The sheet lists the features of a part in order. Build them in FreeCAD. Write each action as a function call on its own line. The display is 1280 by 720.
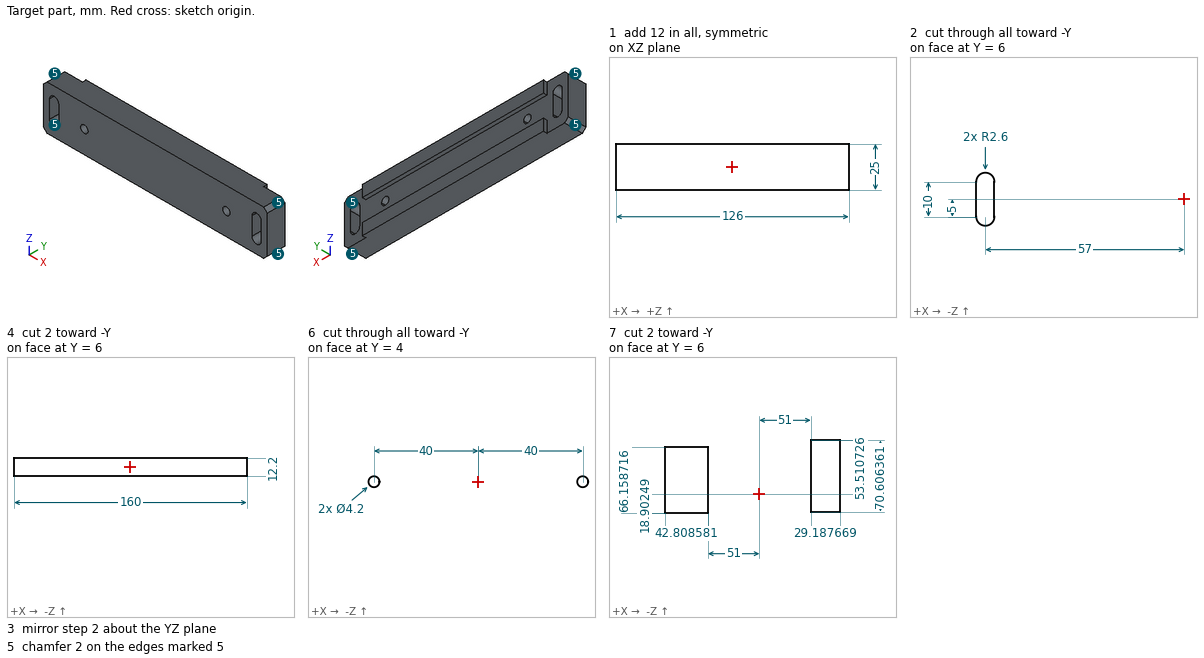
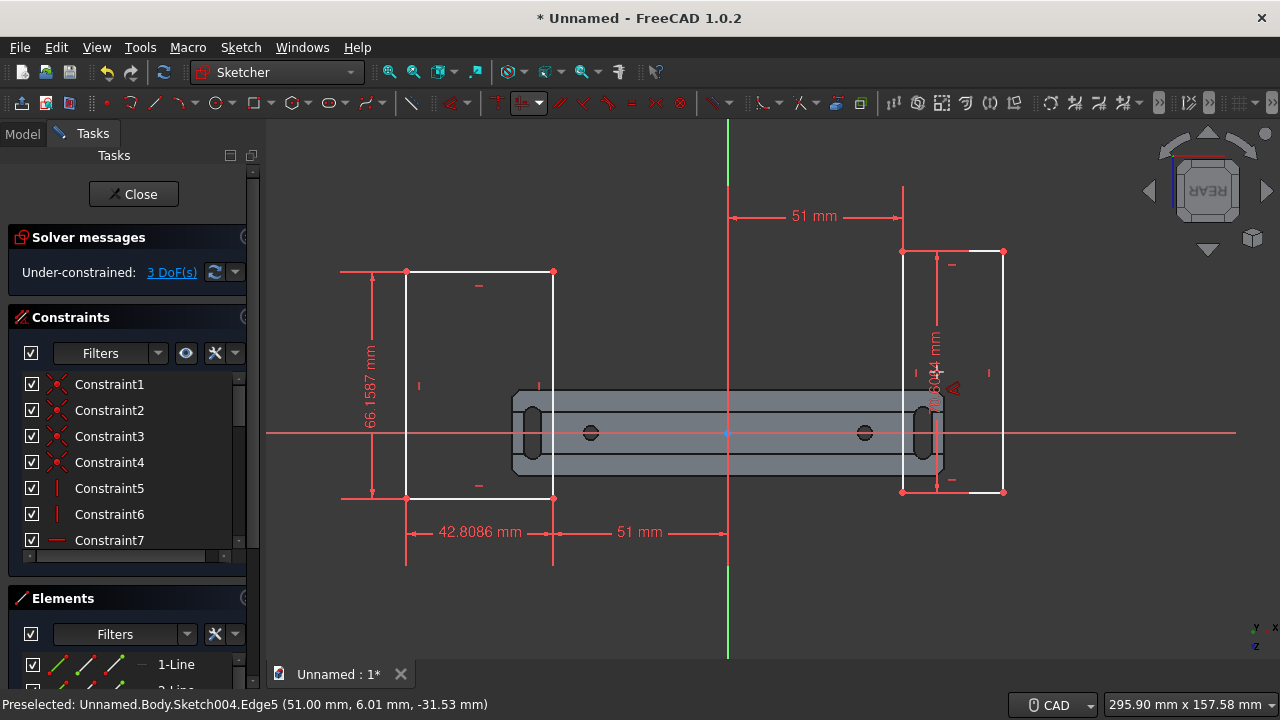
click(933, 493)
click(953, 527)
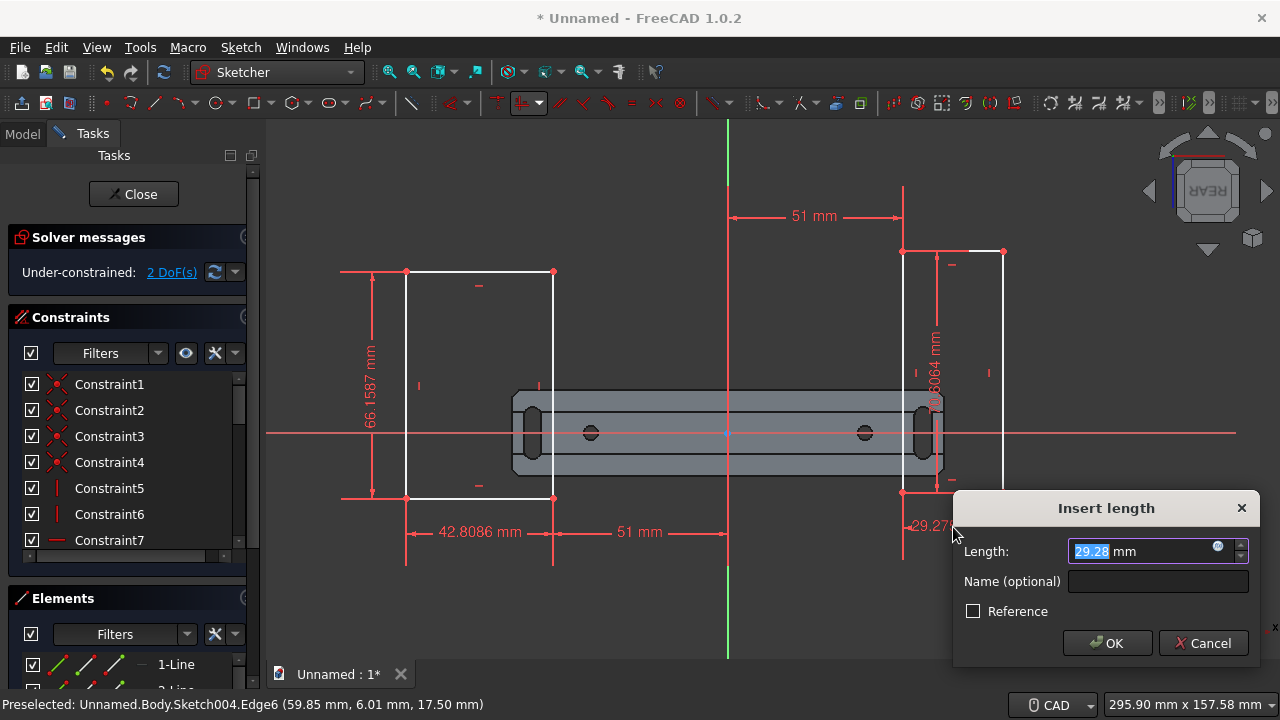
text(29.187669)
key(Return)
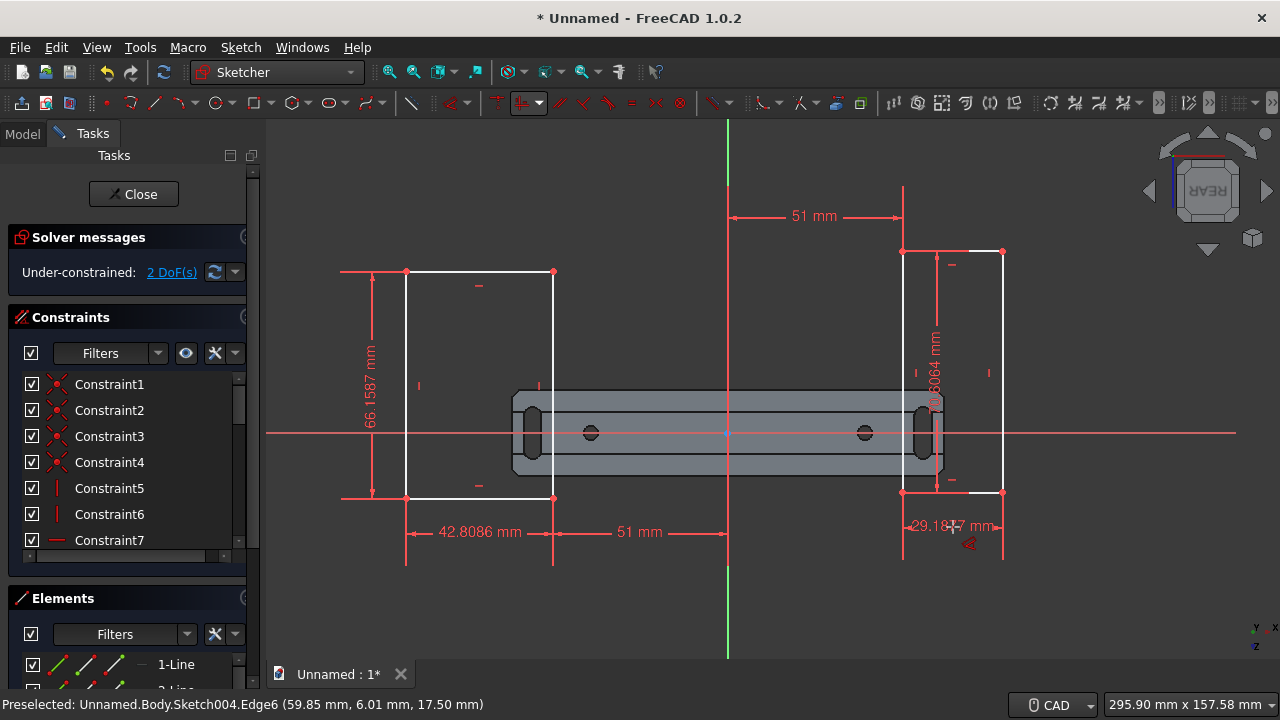
click(406, 499)
click(372, 466)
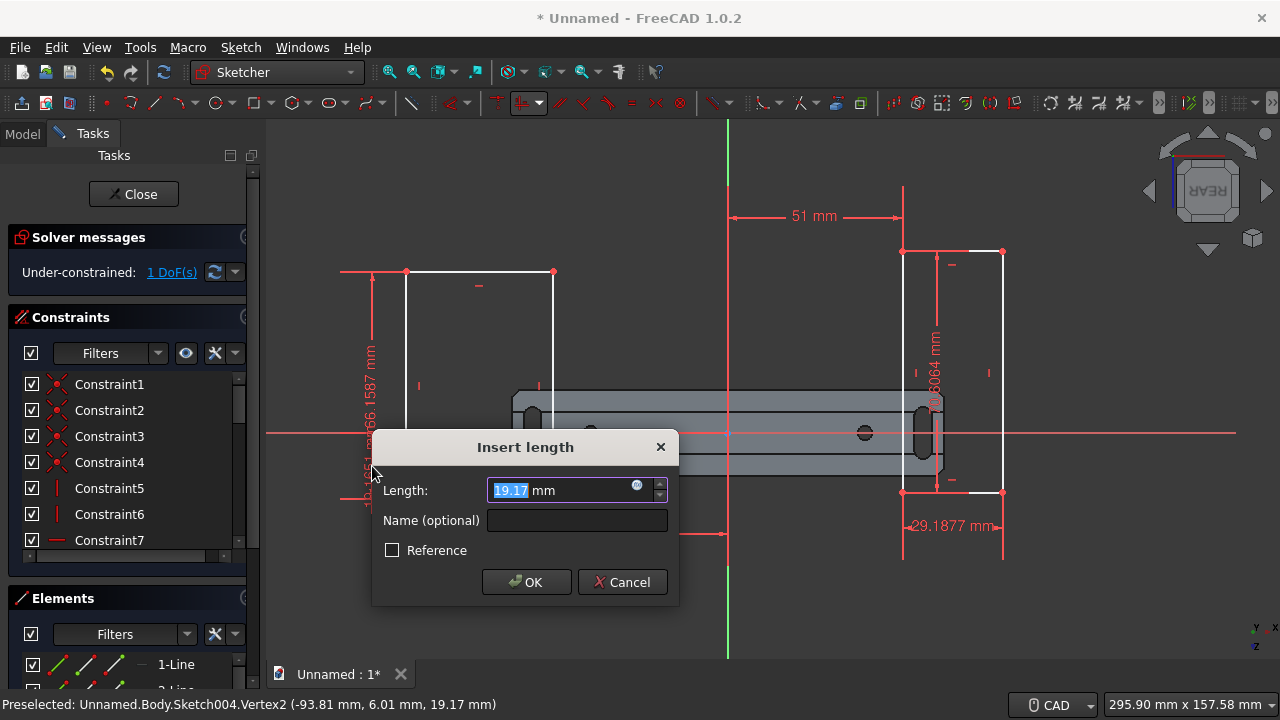
text(18.90249)
key(Return)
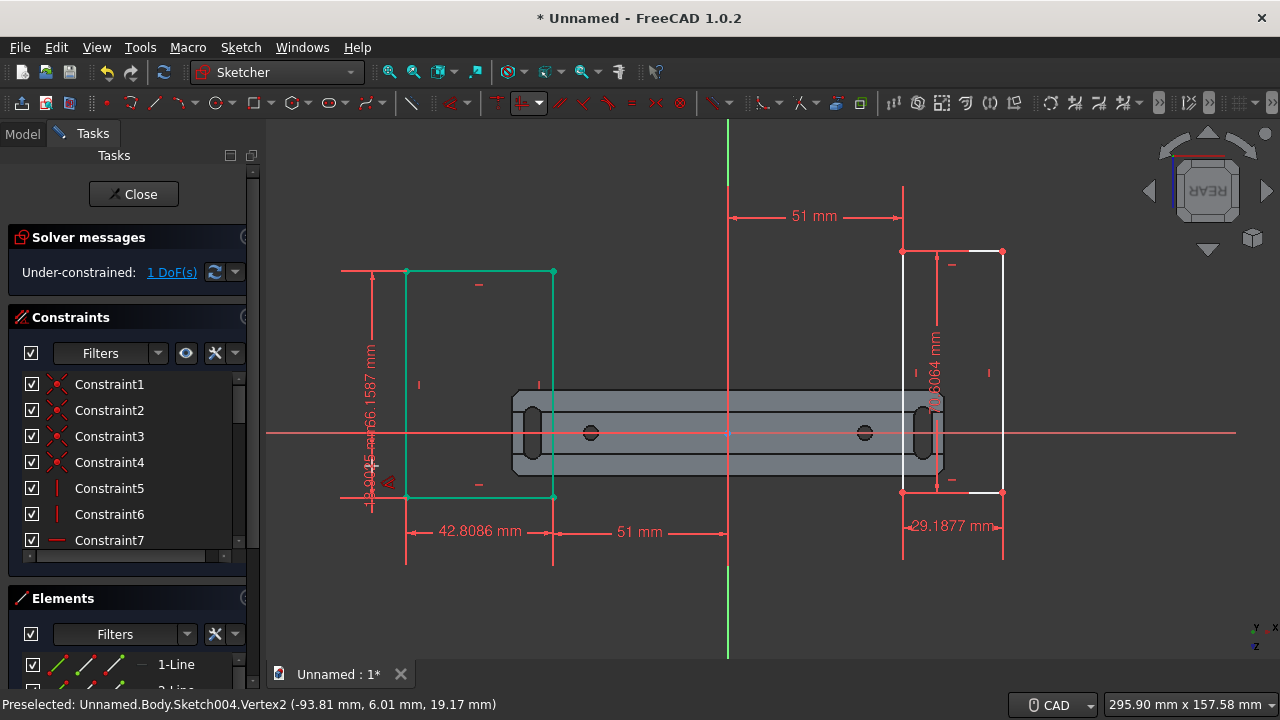
click(903, 251)
click(937, 342)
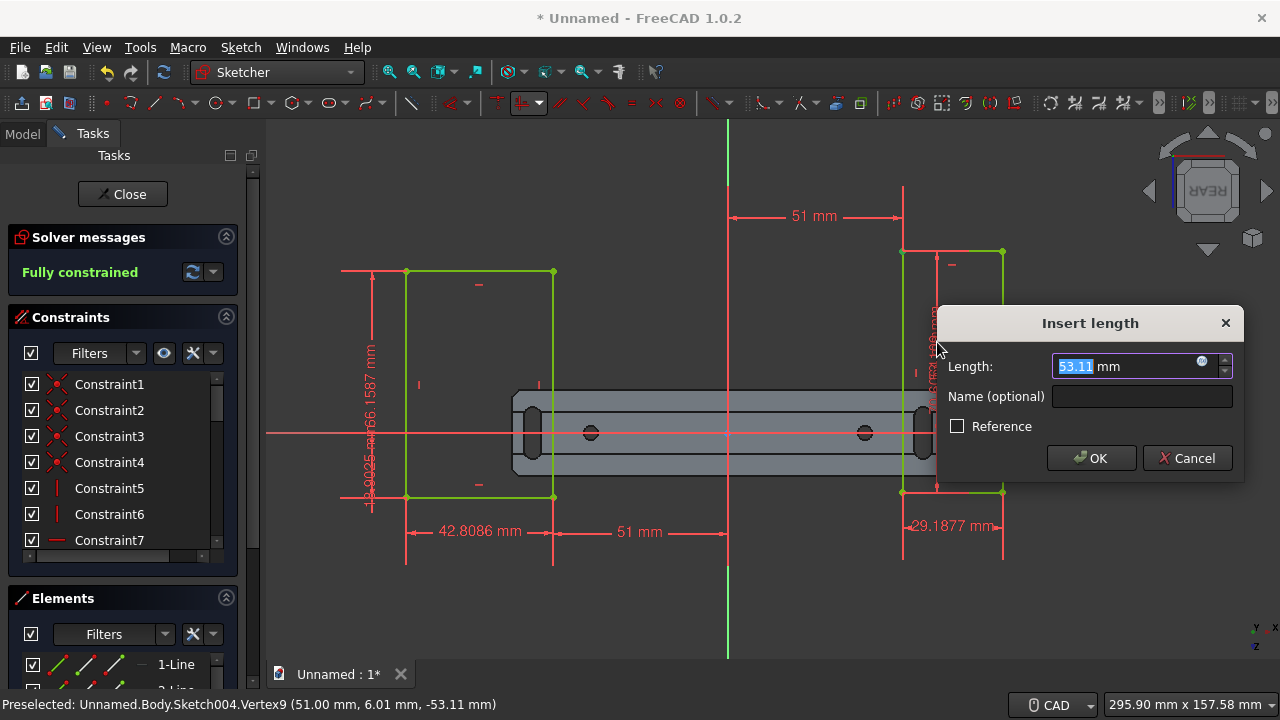
text(53.510726)
key(Return)
key(Escape)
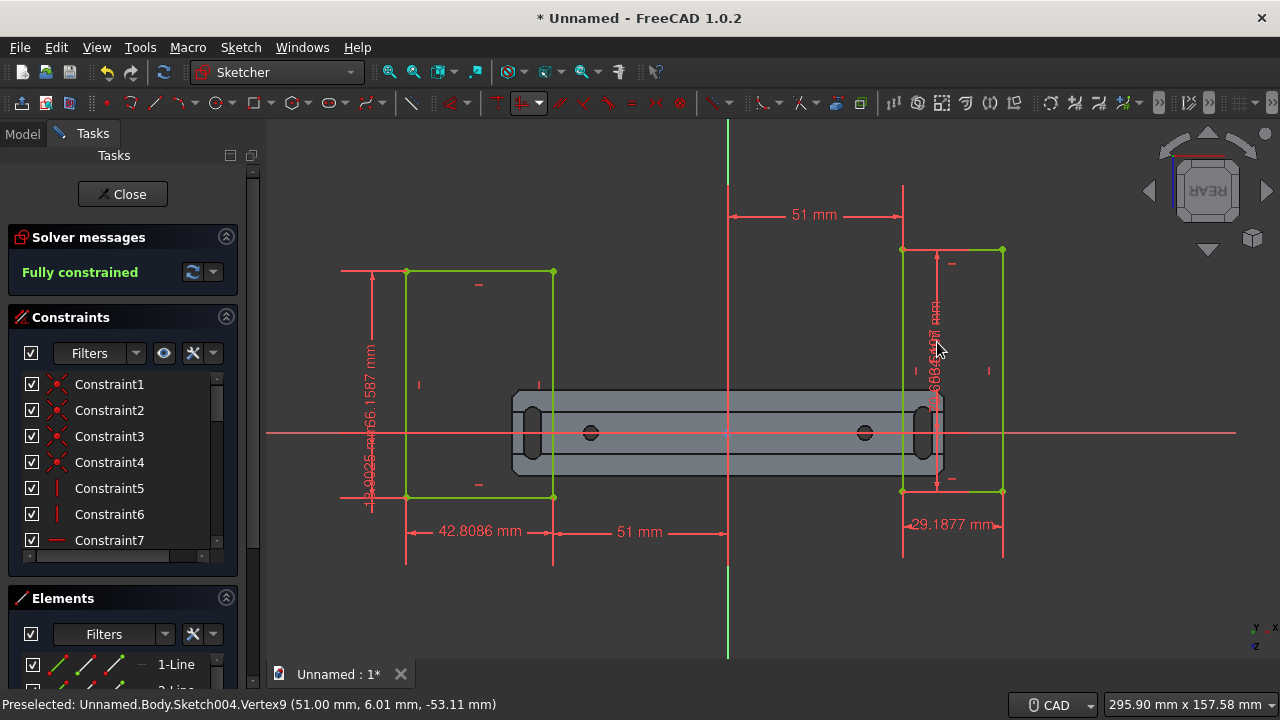
click(123, 194)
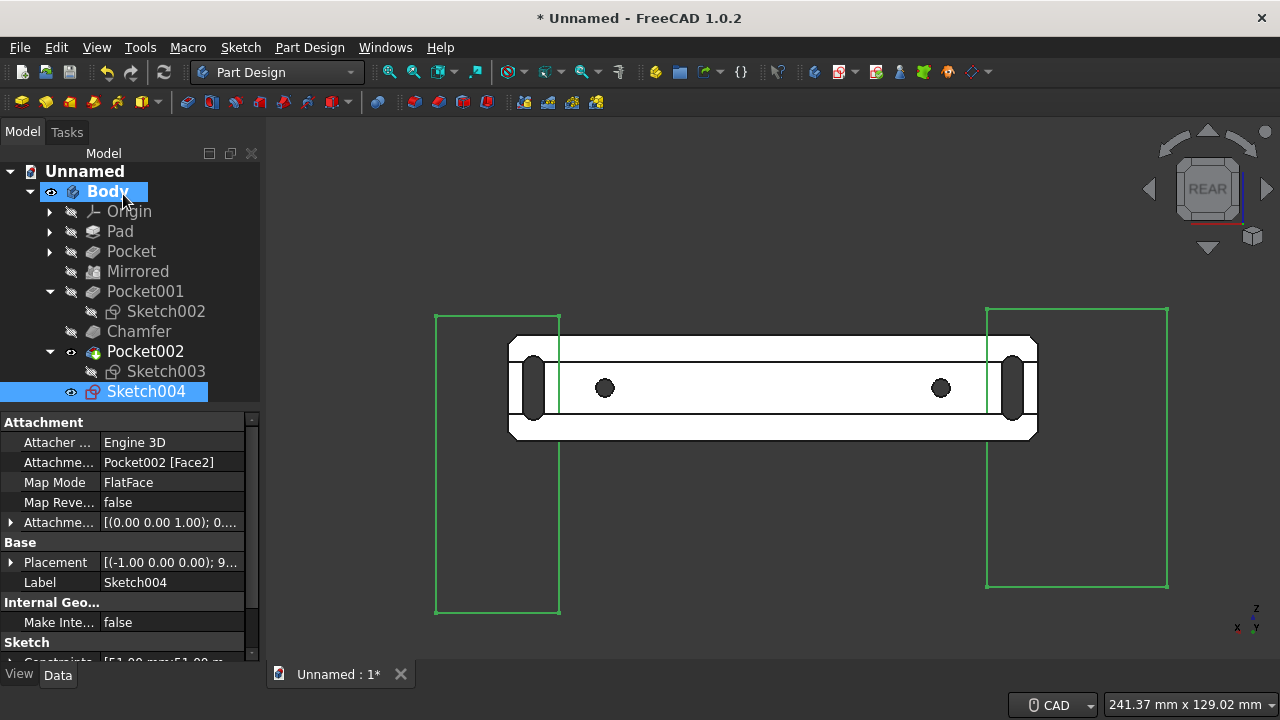
click(188, 102)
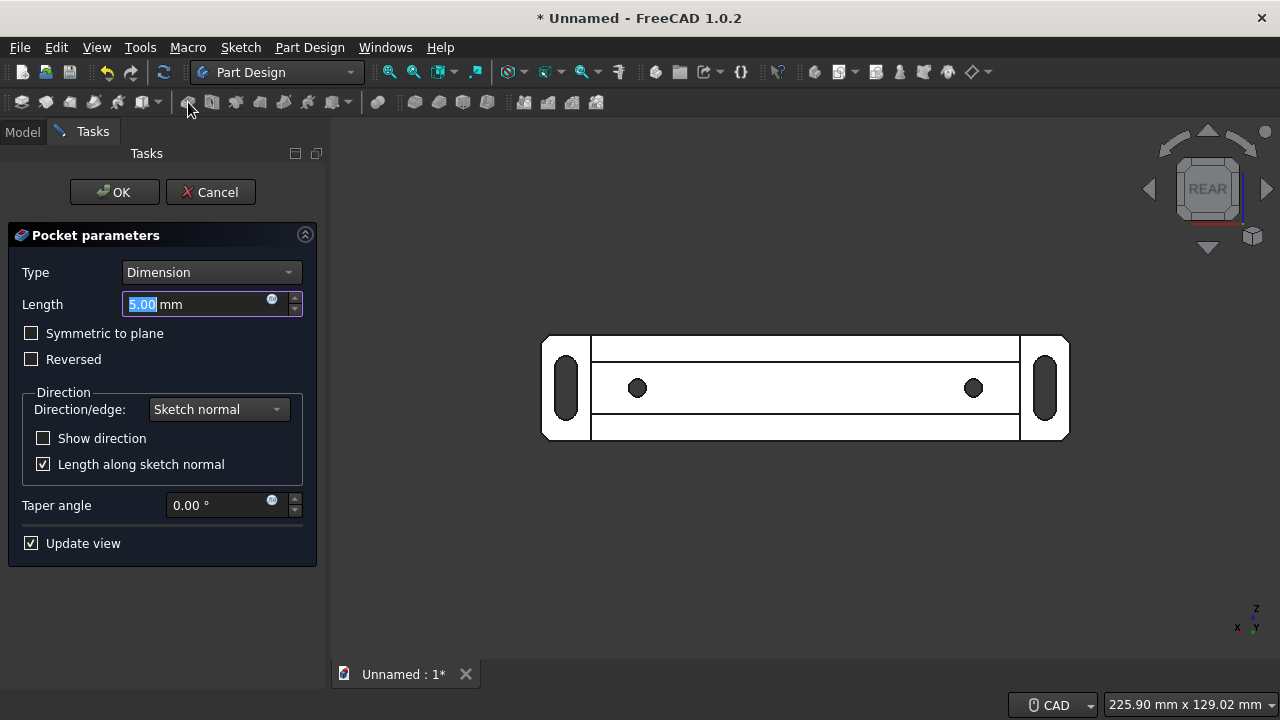
text(2)
key(Tab)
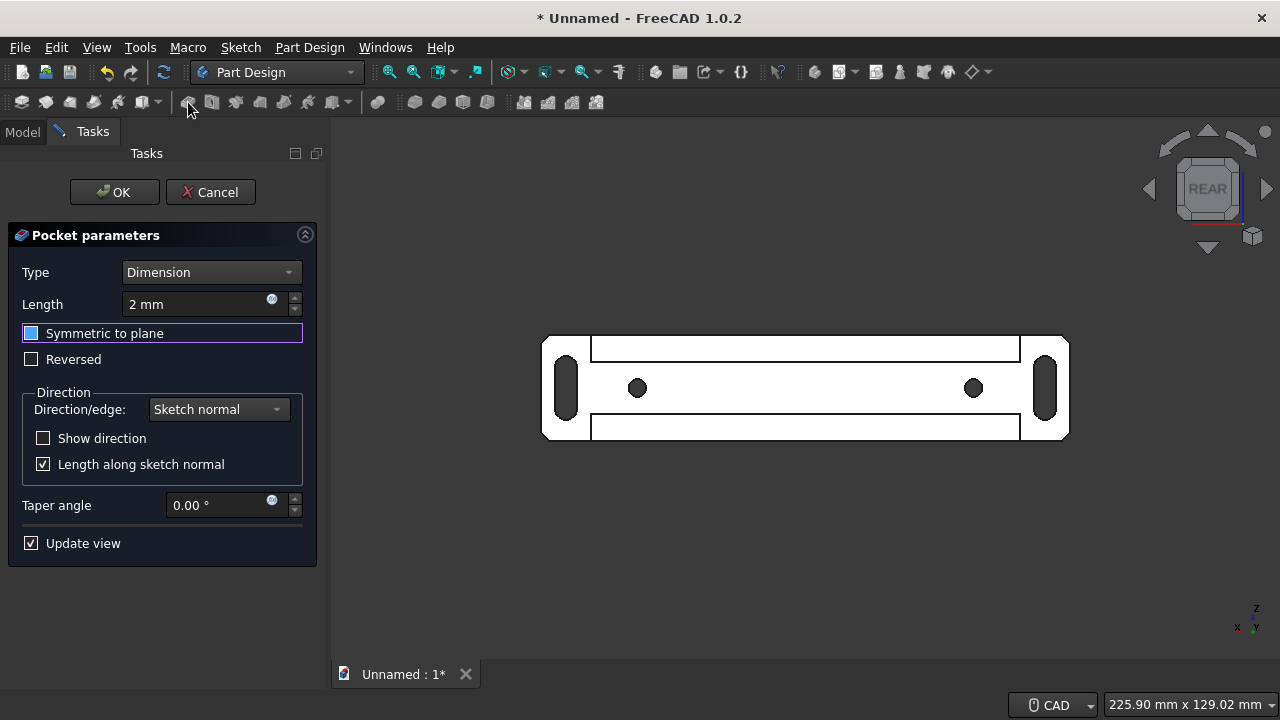
click(115, 192)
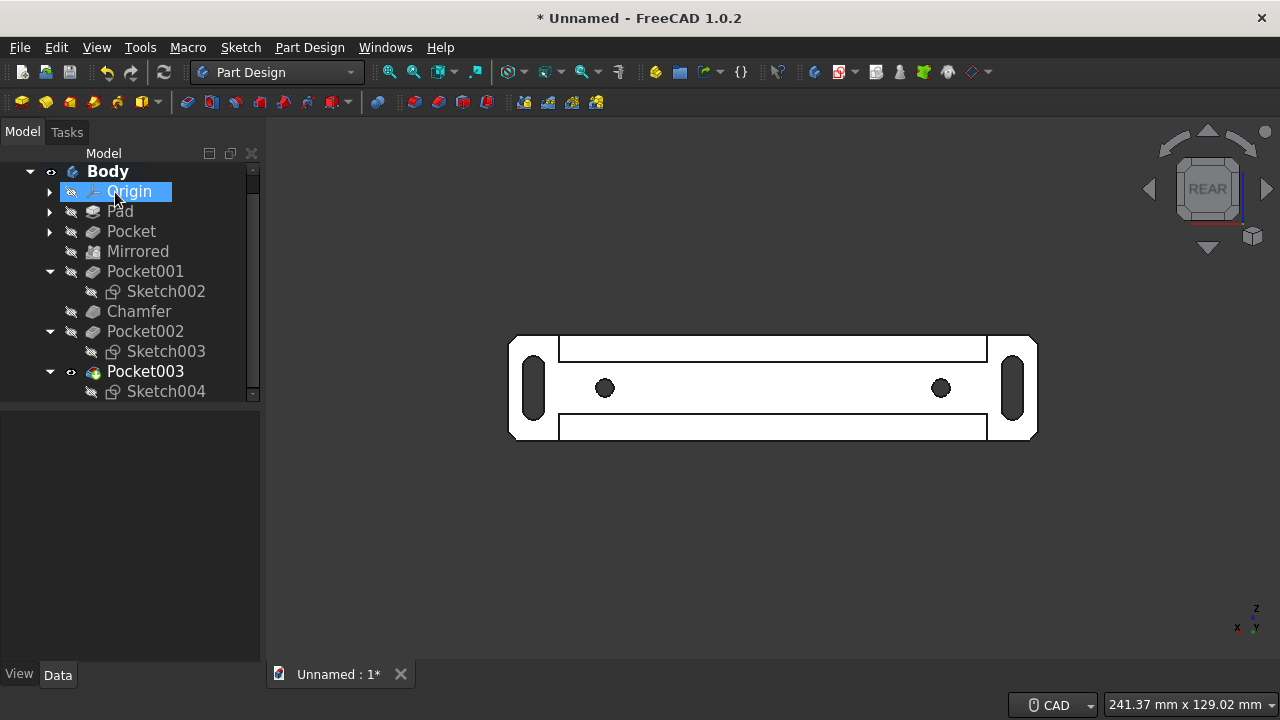
key(0)